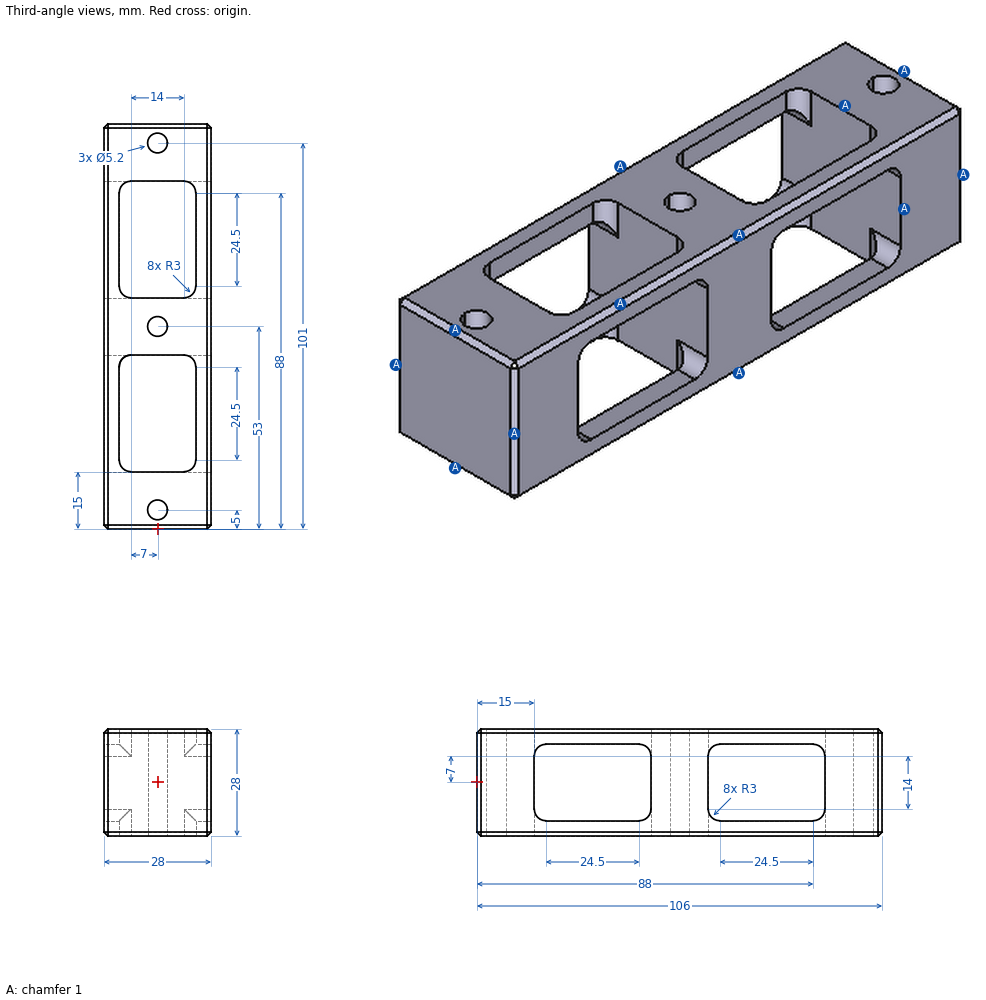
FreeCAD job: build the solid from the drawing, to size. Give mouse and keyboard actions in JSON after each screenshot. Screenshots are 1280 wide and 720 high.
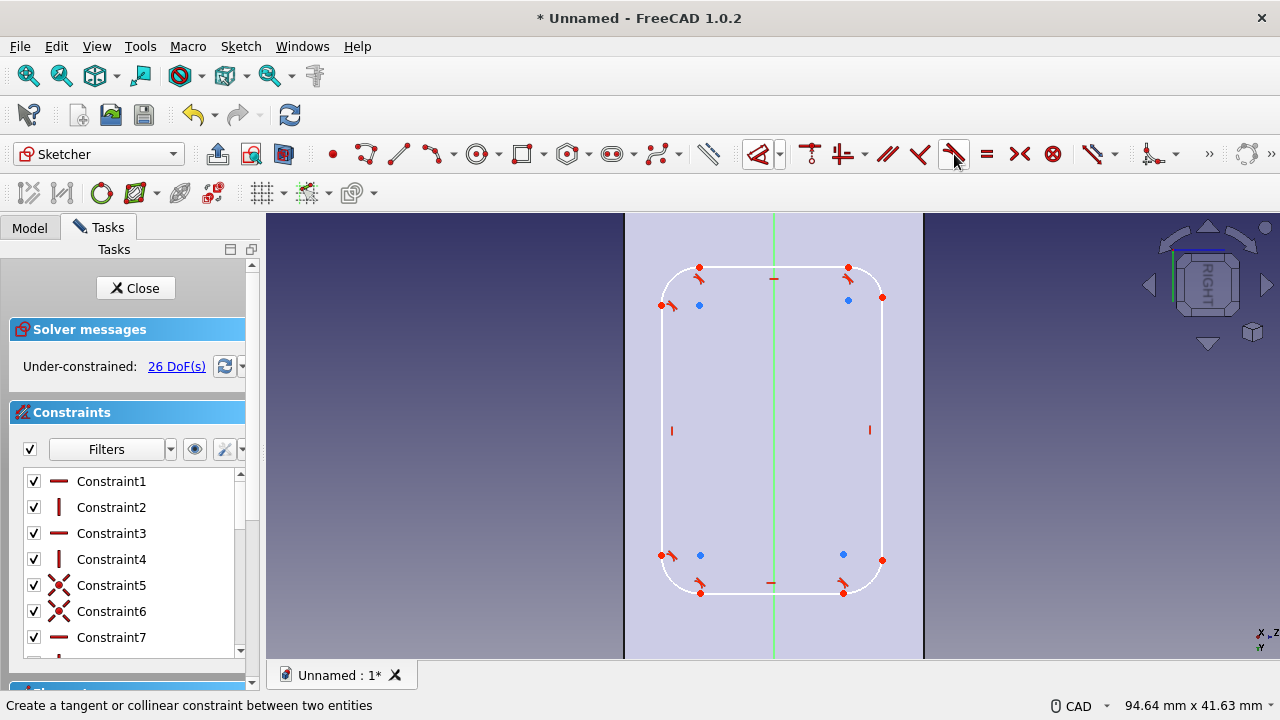
{"action": "left_click", "coordinate": [882, 482]}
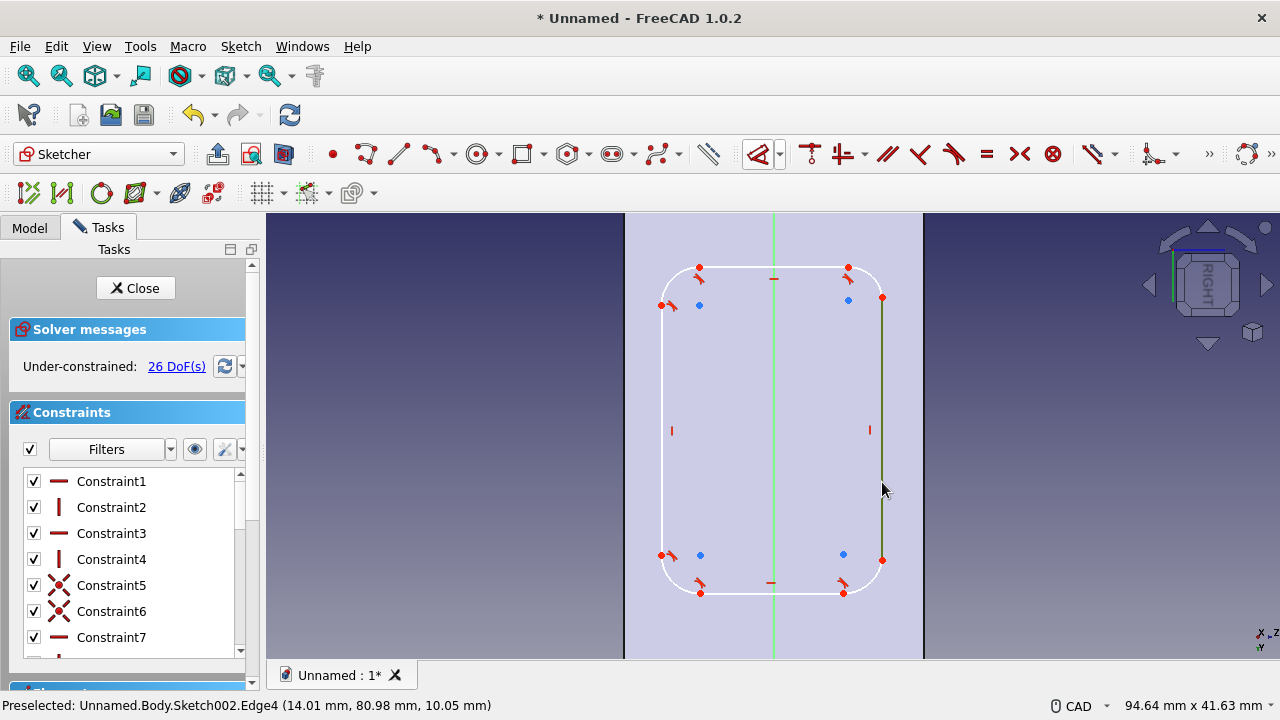
{"action": "left_click", "coordinate": [859, 590]}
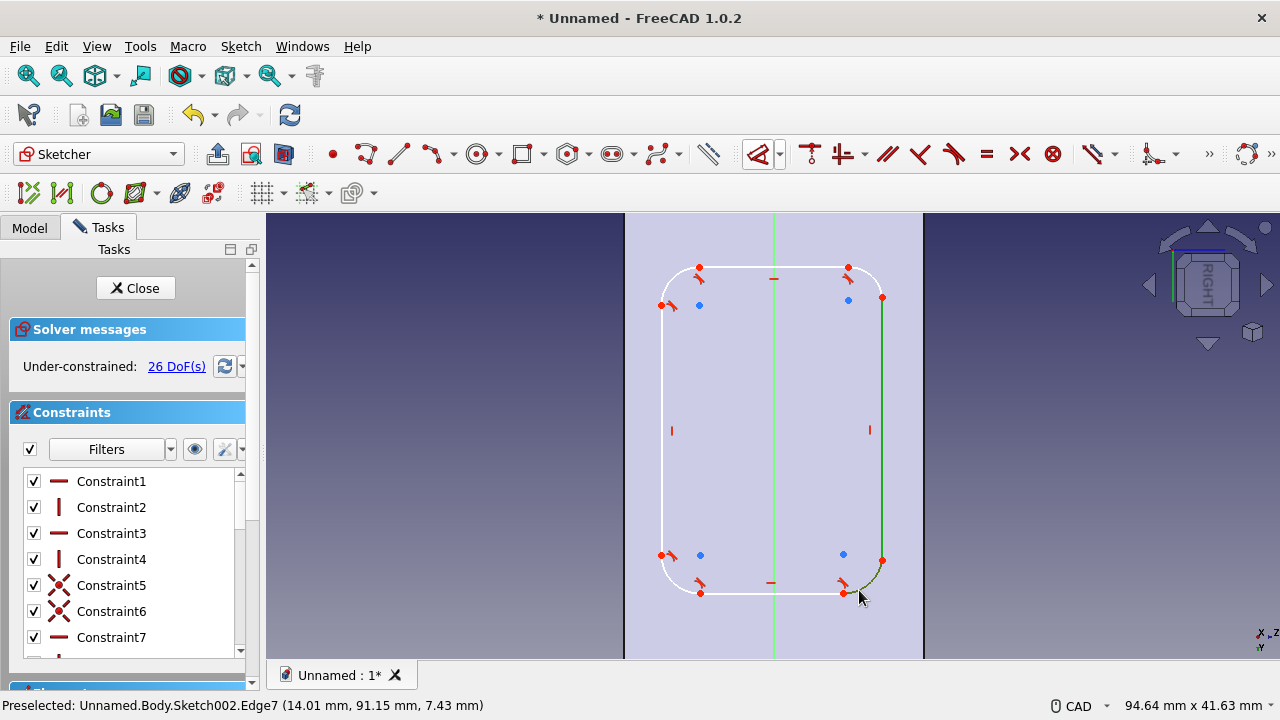
{"action": "left_click", "coordinate": [954, 154]}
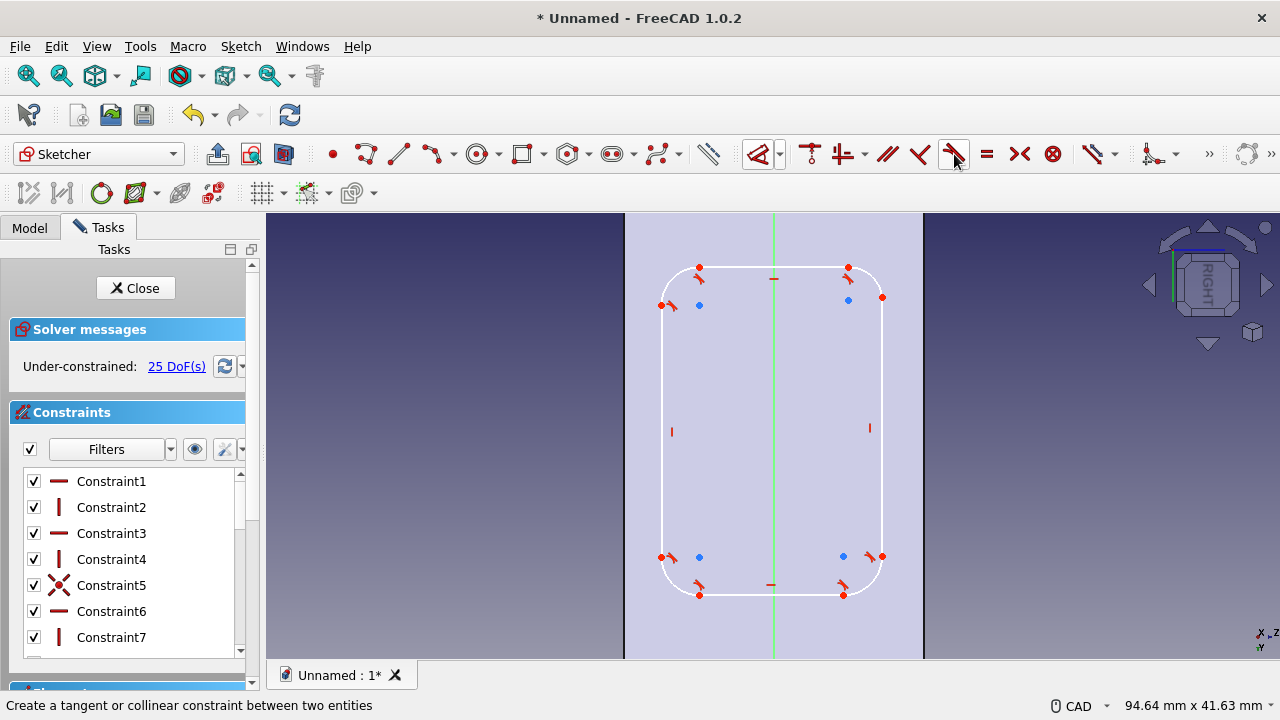
{"action": "left_click", "coordinate": [882, 479]}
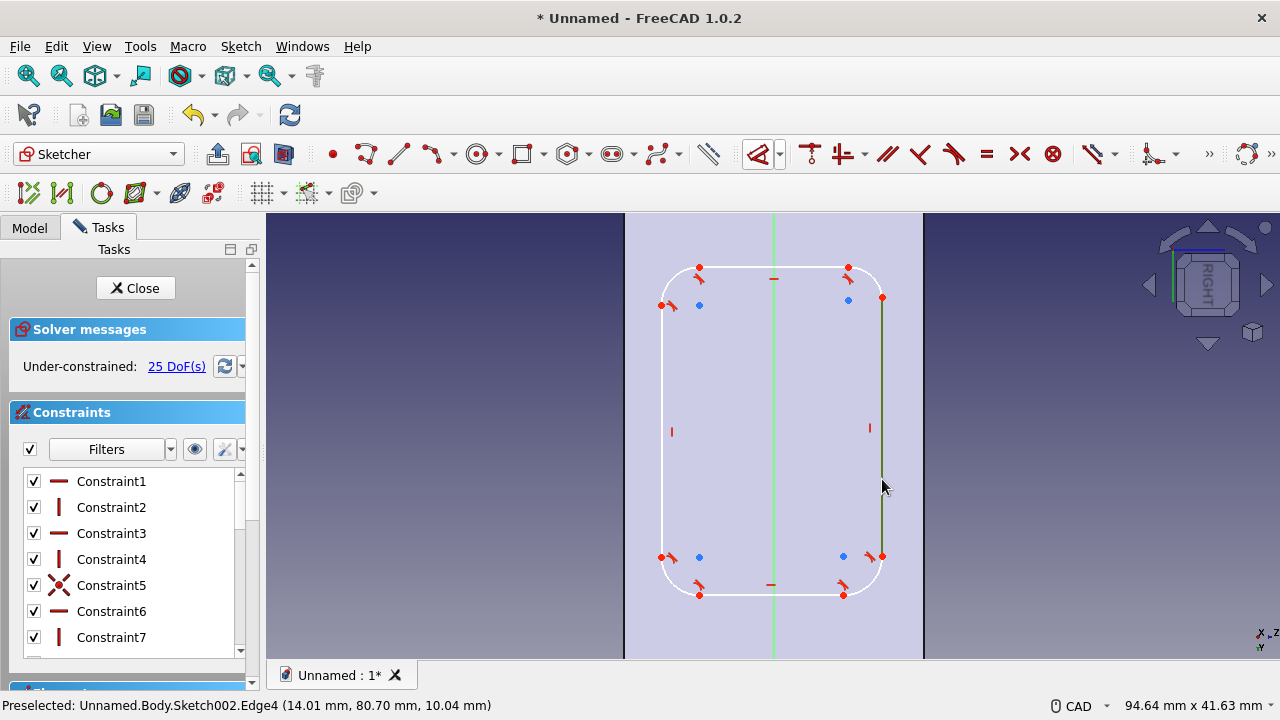
{"action": "left_click", "coordinate": [878, 284]}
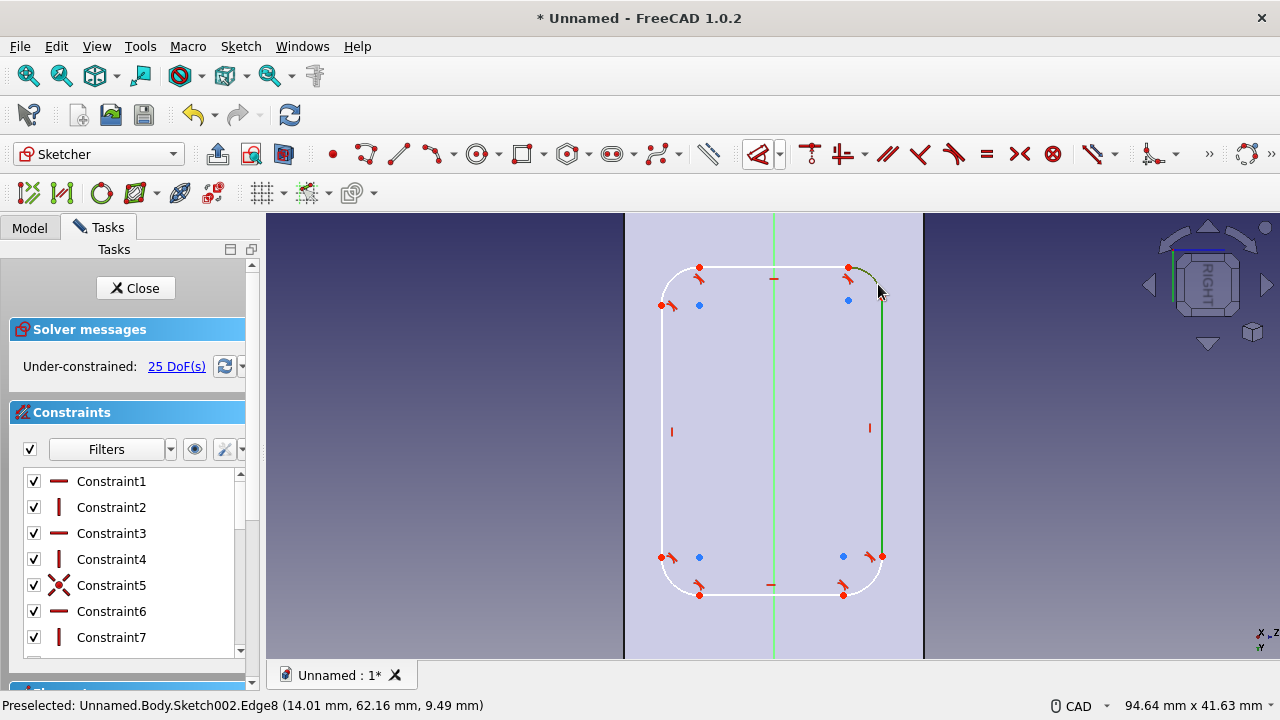
{"action": "key", "text": "t"}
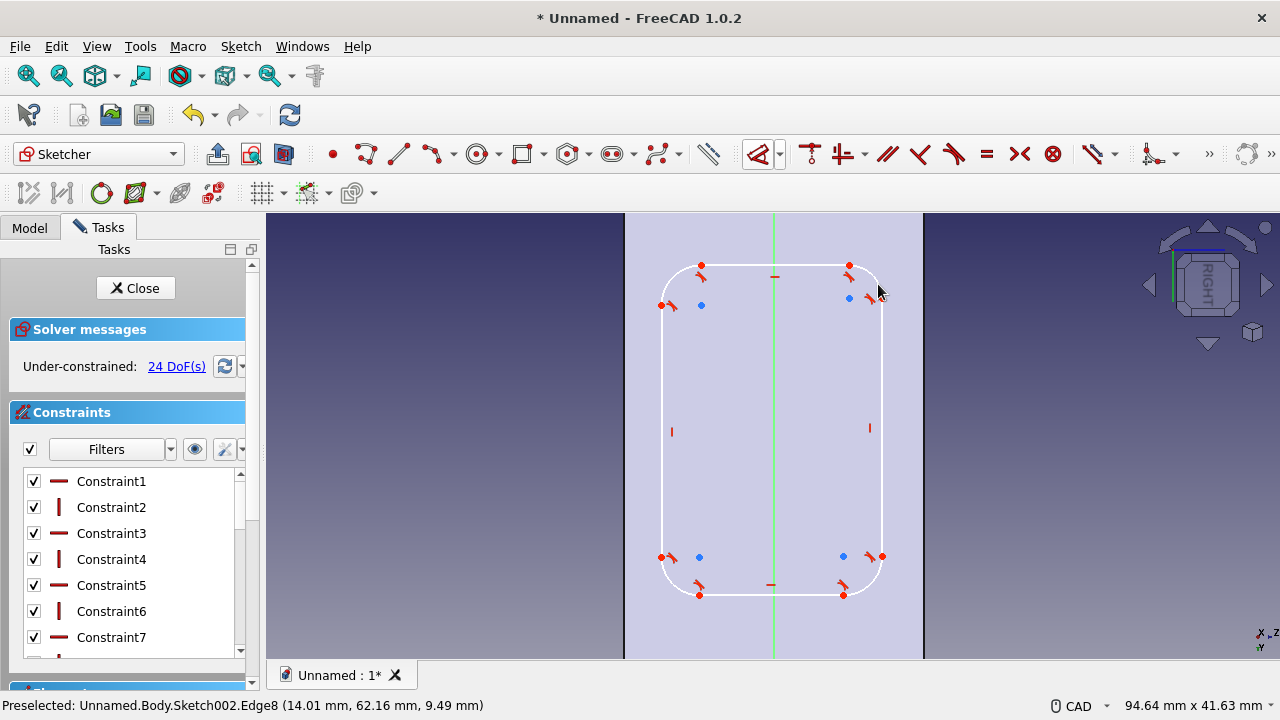
{"action": "scroll", "coordinate": [674, 580], "scroll_direction": "down", "scroll_amount": 6}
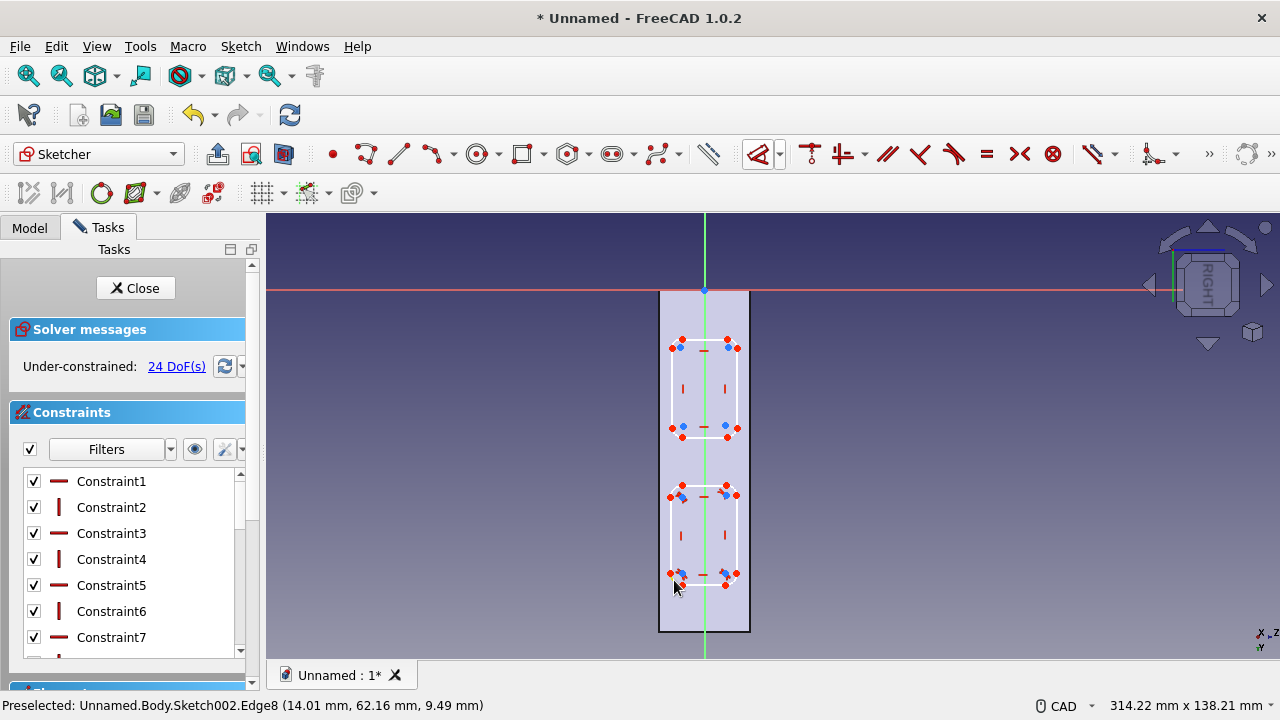
{"action": "scroll", "coordinate": [714, 340], "scroll_direction": "up", "scroll_amount": 3}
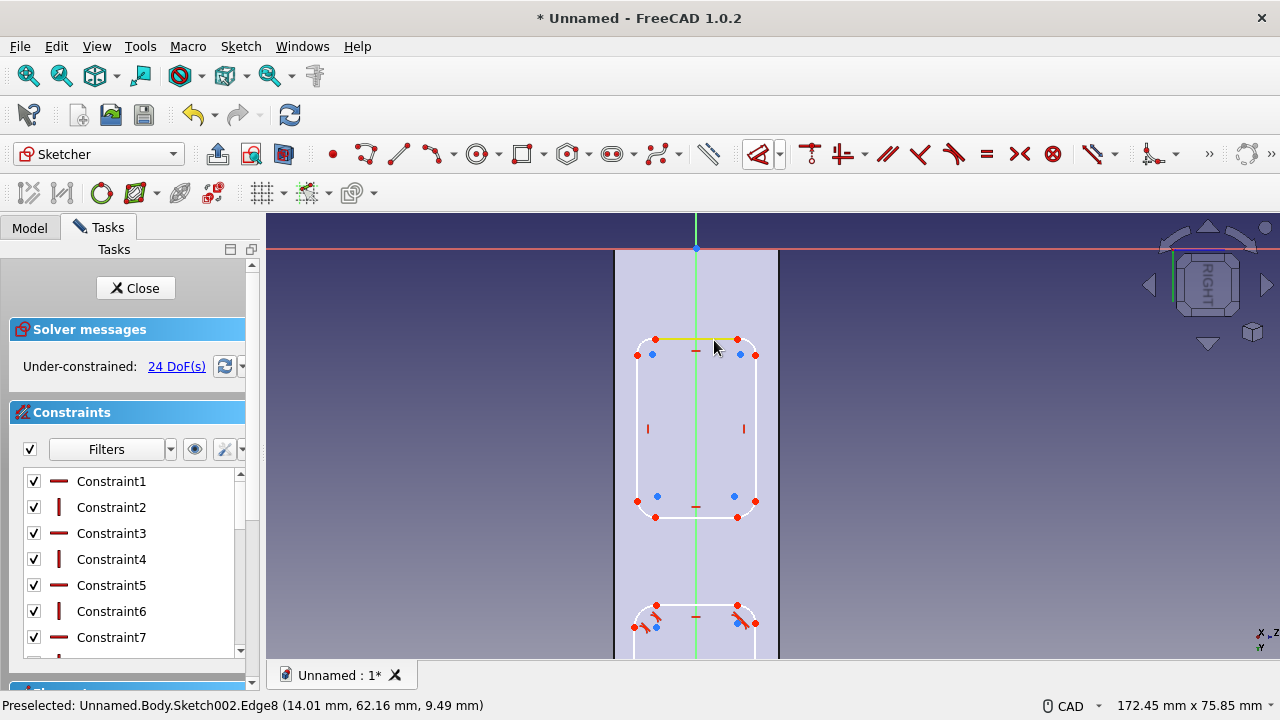
{"action": "left_click", "coordinate": [713, 339]}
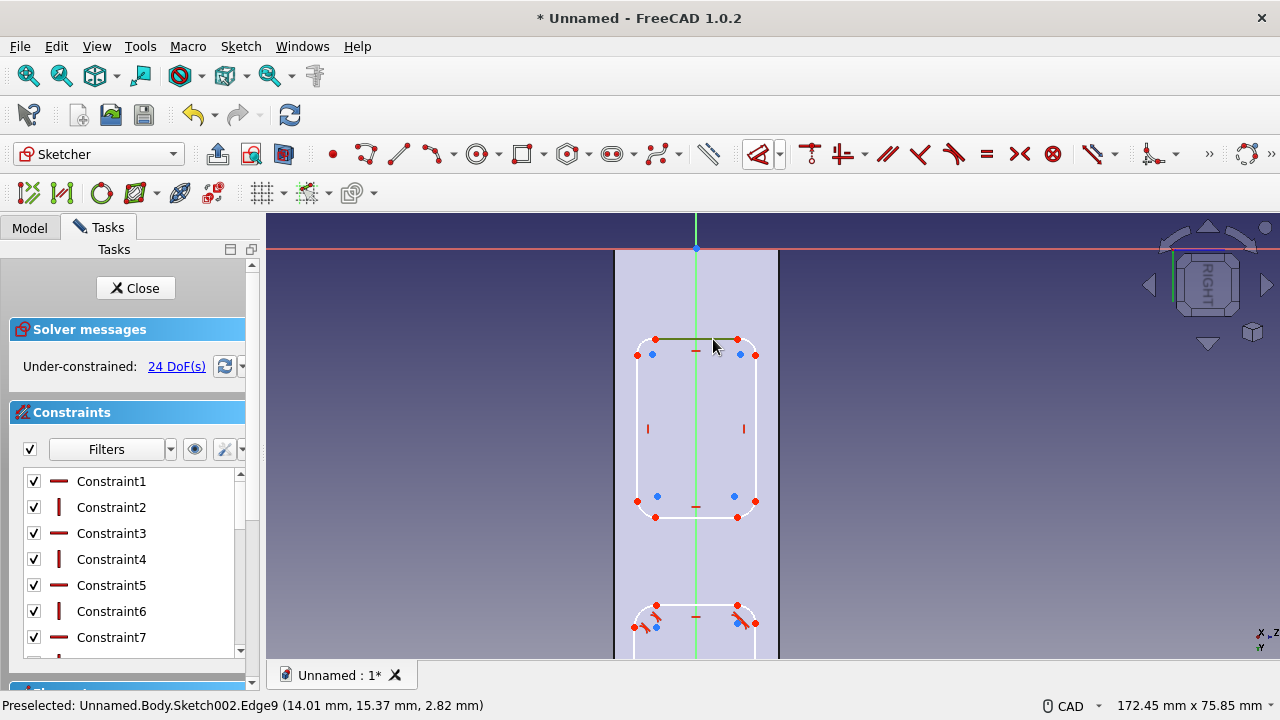
{"action": "left_click", "coordinate": [642, 343]}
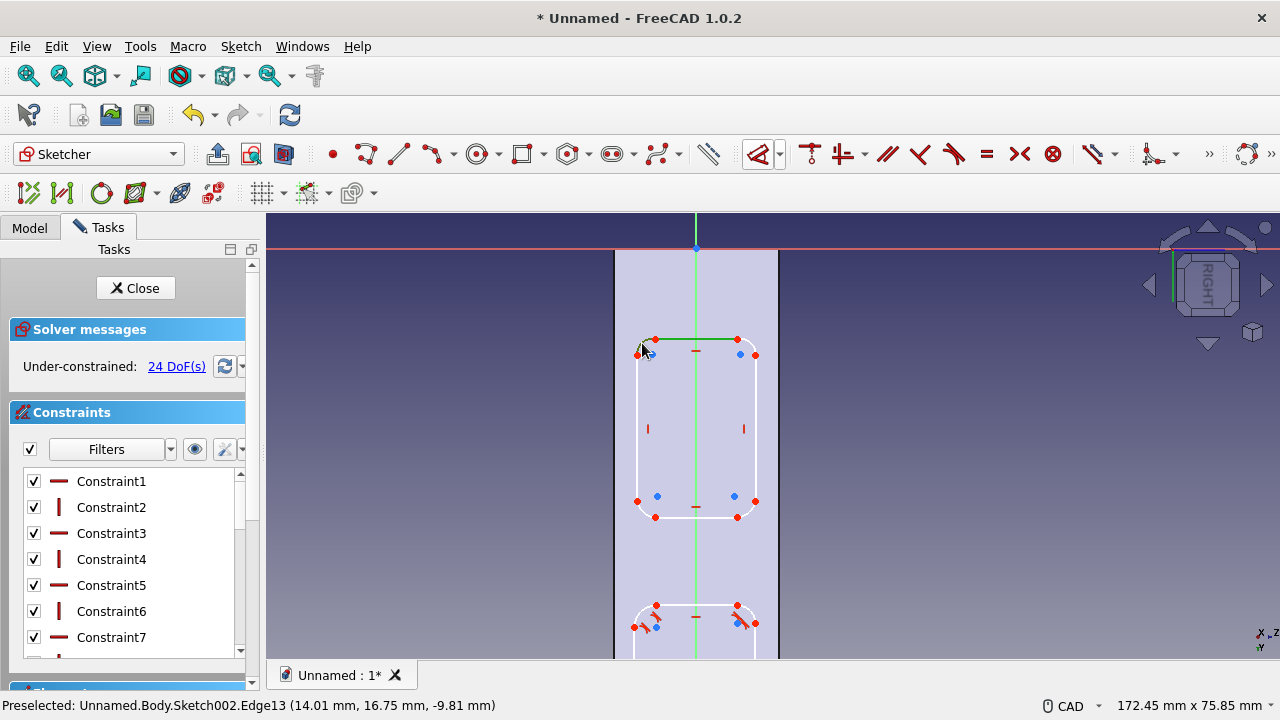
{"action": "left_click", "coordinate": [954, 154]}